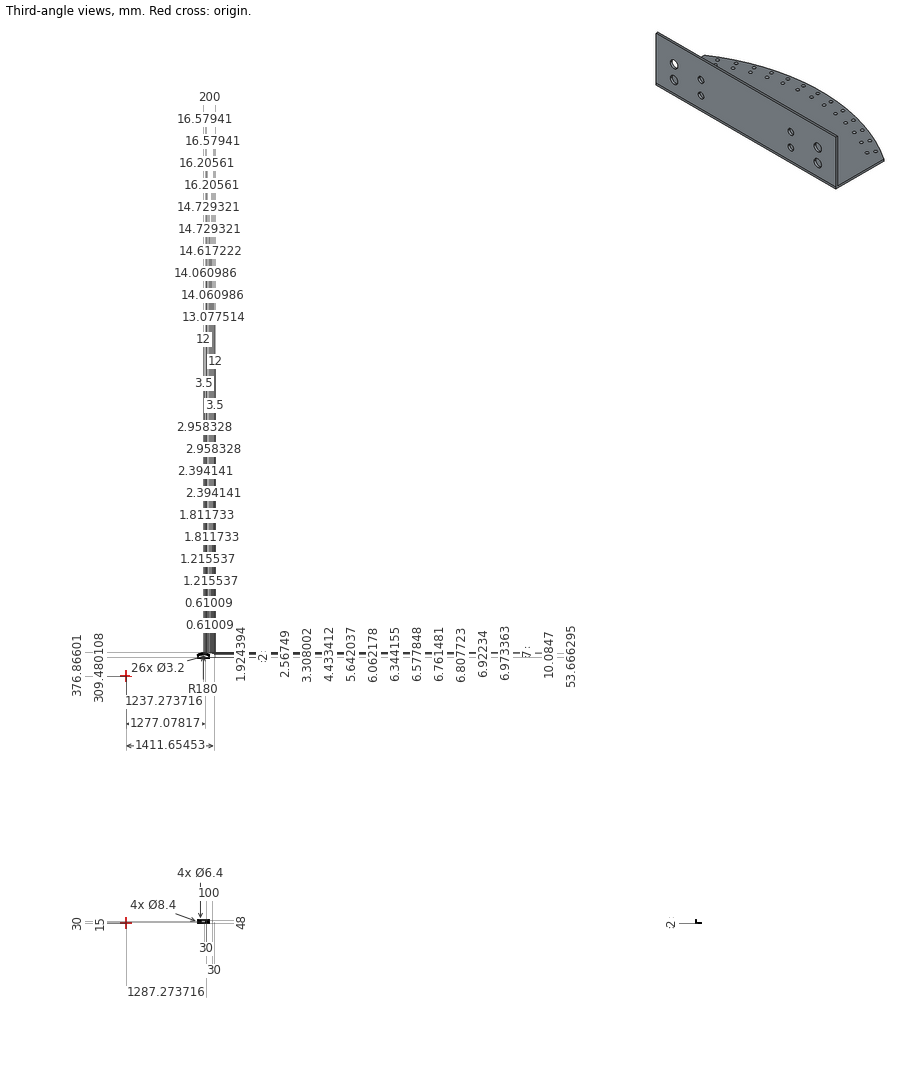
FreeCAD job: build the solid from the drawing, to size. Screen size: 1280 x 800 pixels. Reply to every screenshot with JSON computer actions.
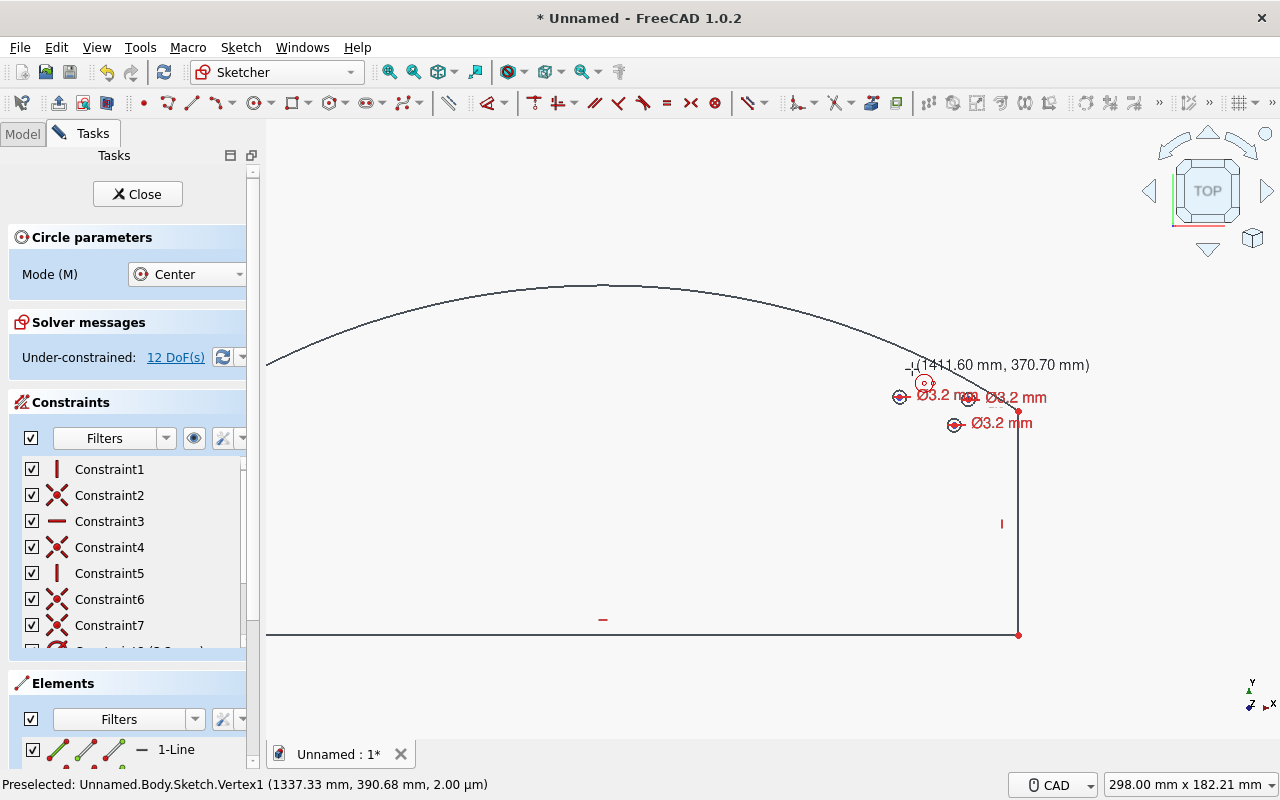
{"action": "left_click", "coordinate": [912, 369]}
{"action": "mouse_move", "coordinate": [907, 364]}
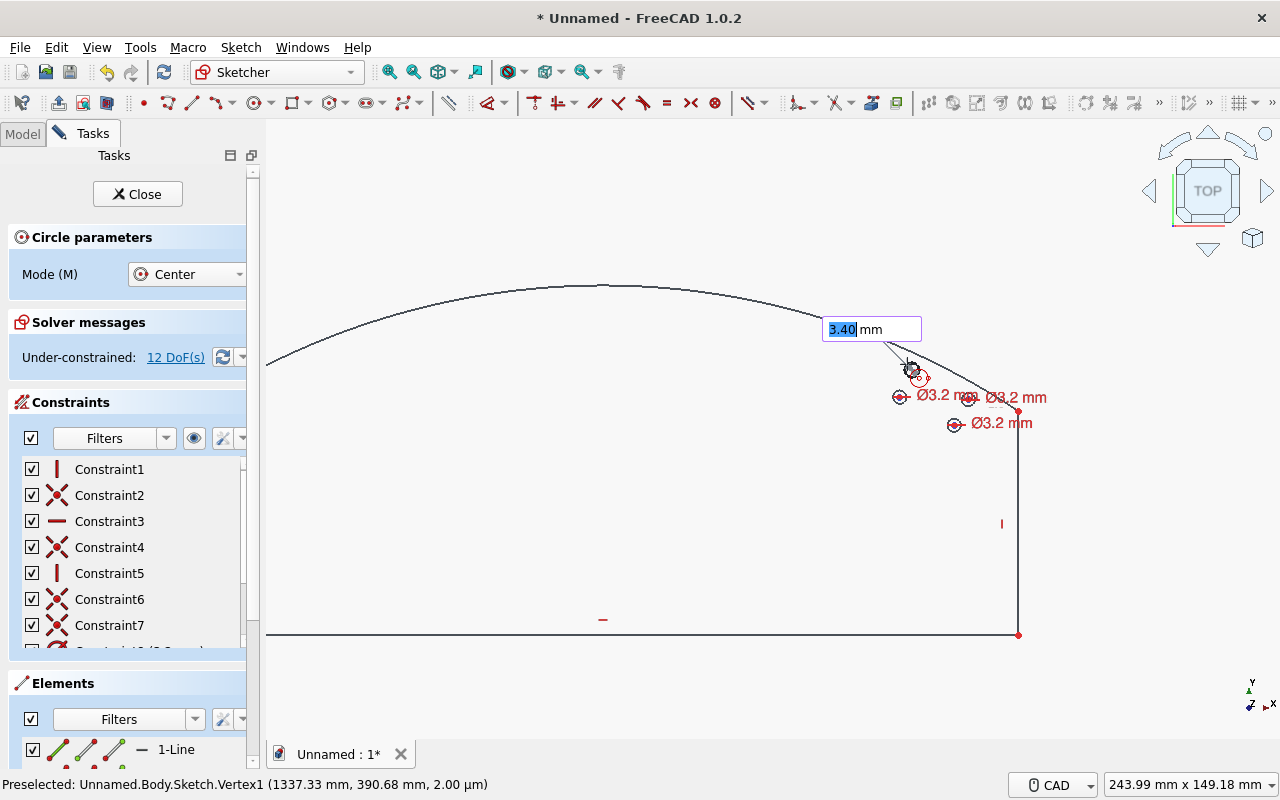
{"action": "type", "text": "3.2"}
{"action": "key", "text": "Return"}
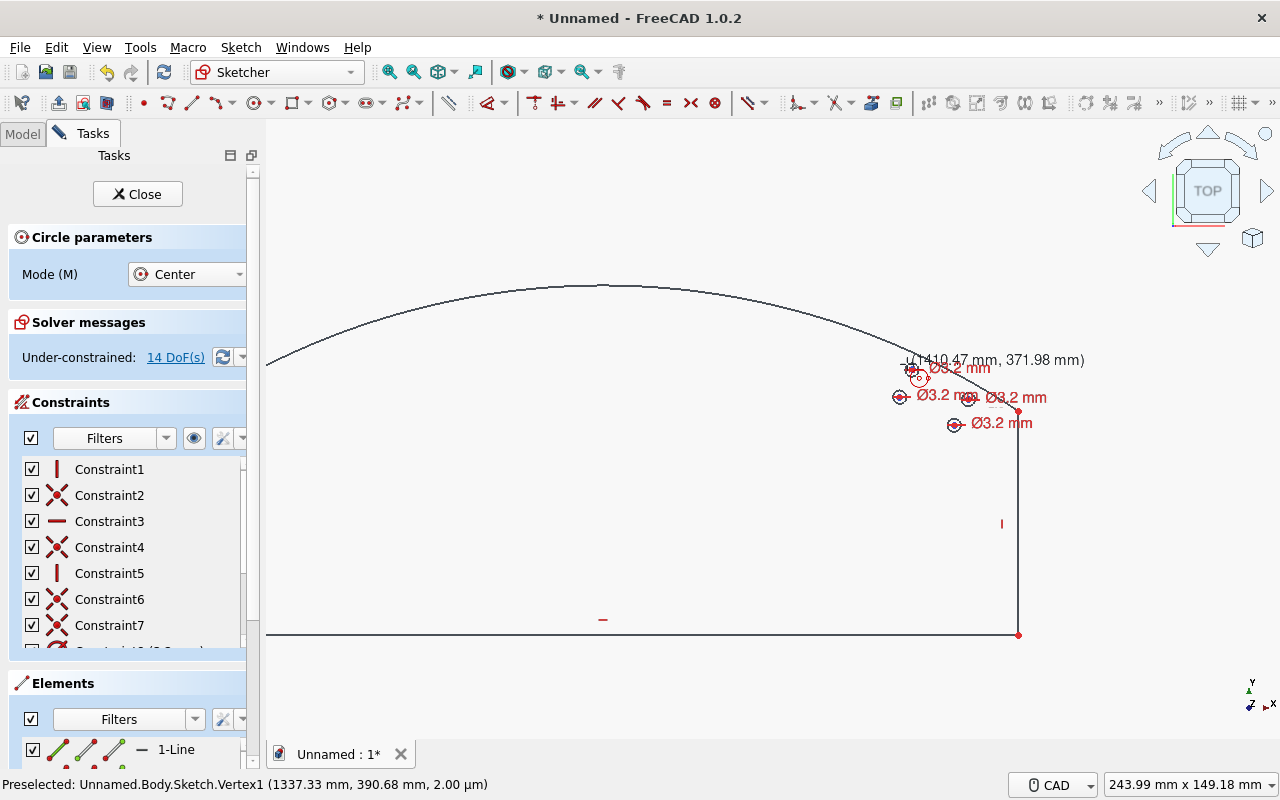
{"action": "scroll", "coordinate": [843, 372], "scroll_direction": "up", "scroll_amount": 7}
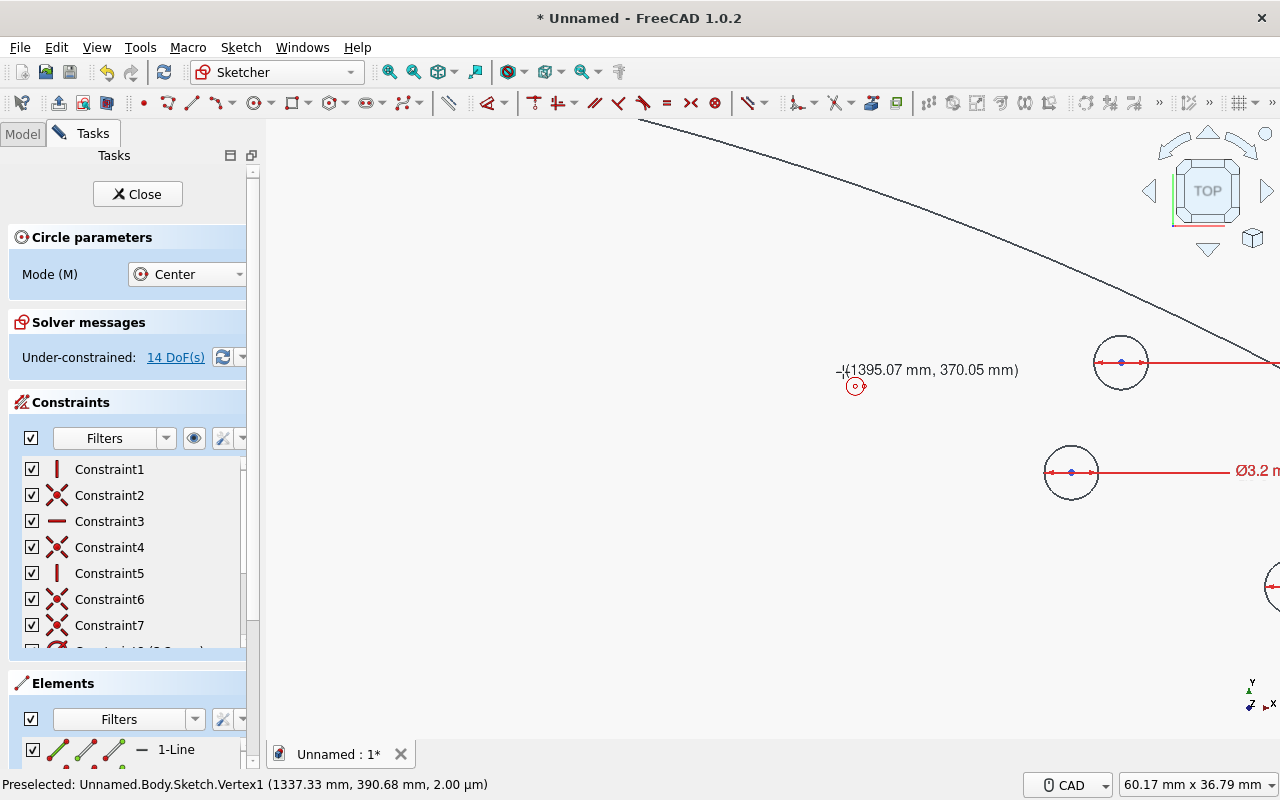
{"action": "scroll", "coordinate": [870, 371], "scroll_direction": "down", "scroll_amount": 9}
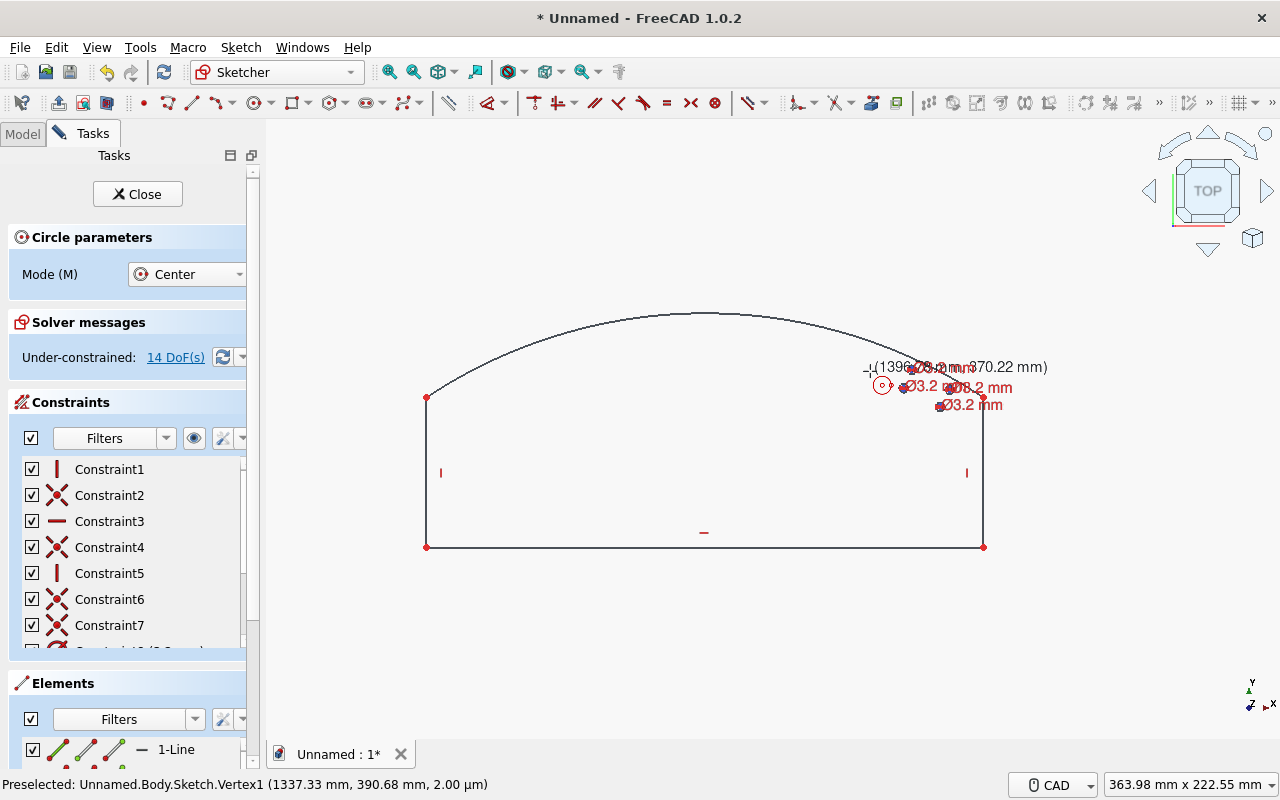
{"action": "left_click", "coordinate": [866, 371]}
{"action": "mouse_move", "coordinate": [869, 368]}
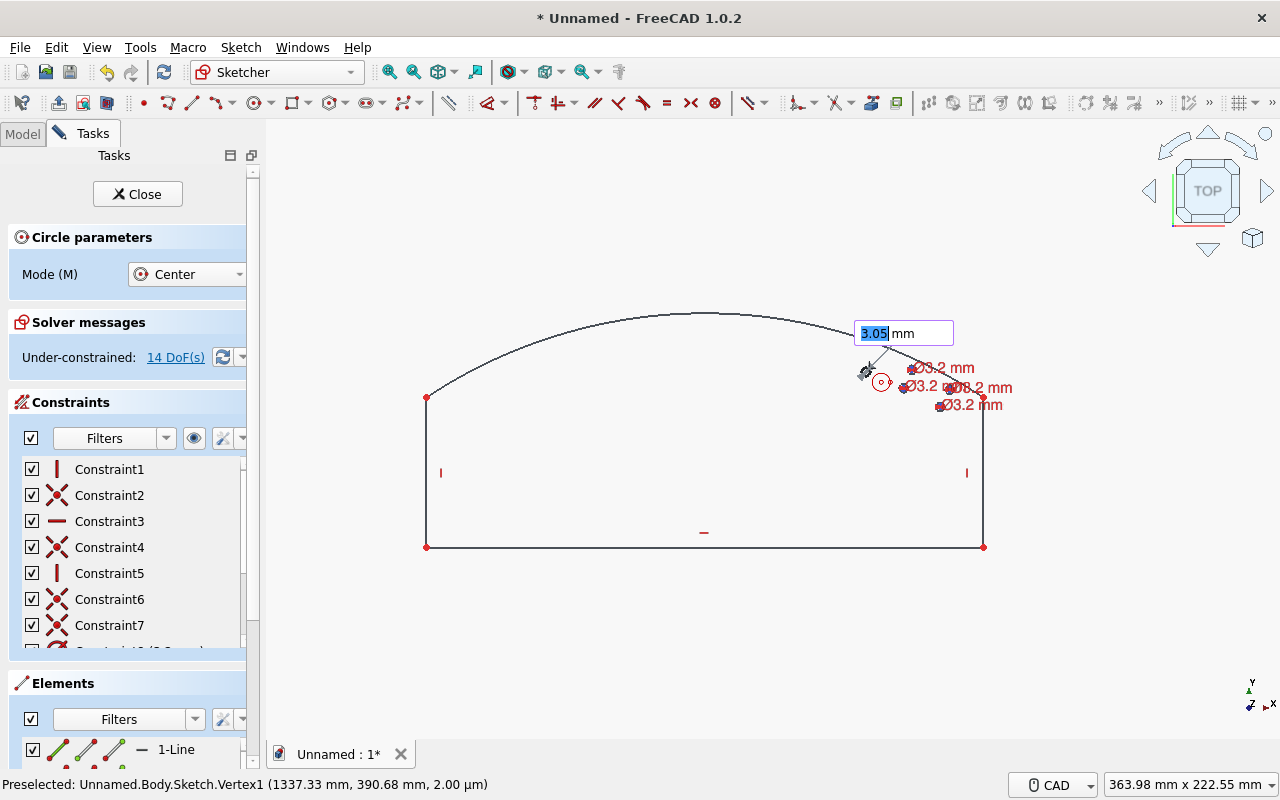
{"action": "type", "text": "3.2"}
{"action": "key", "text": "Return"}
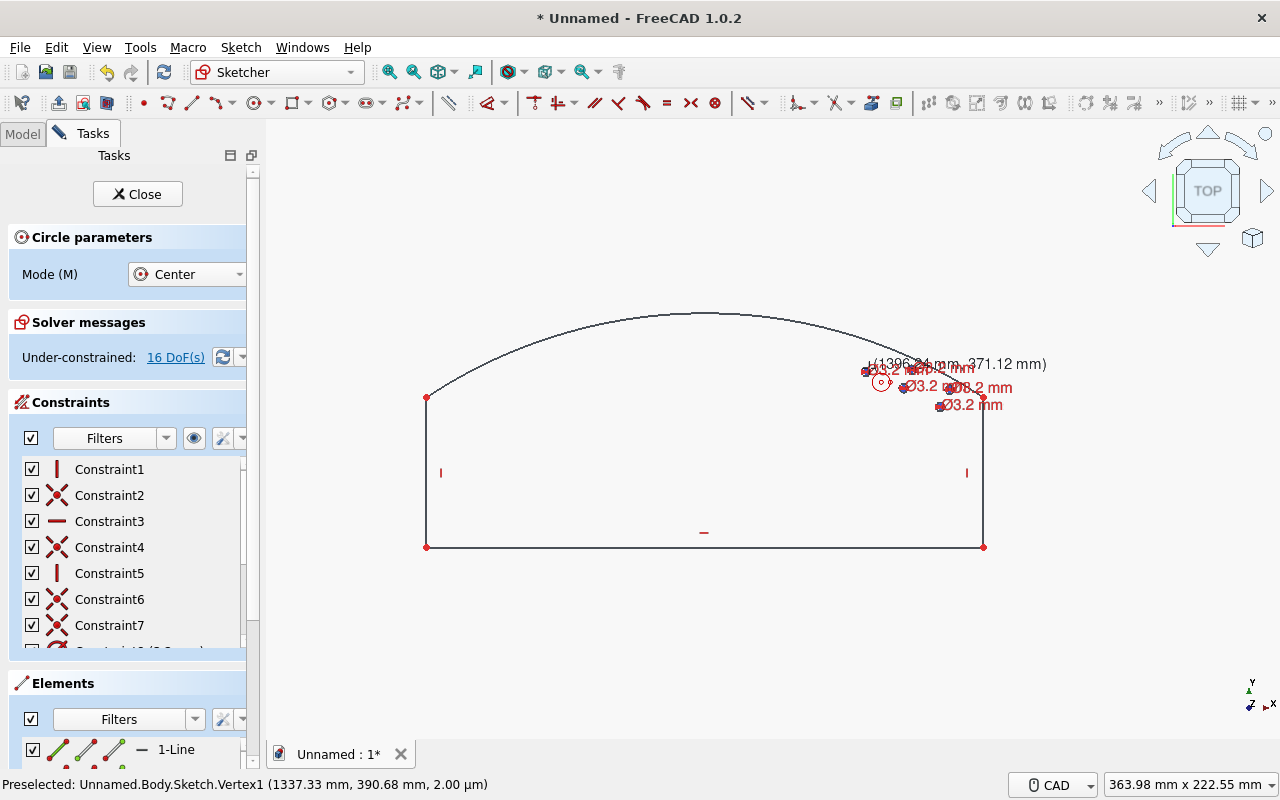
{"action": "scroll", "coordinate": [469, 406], "scroll_direction": "up", "scroll_amount": 9}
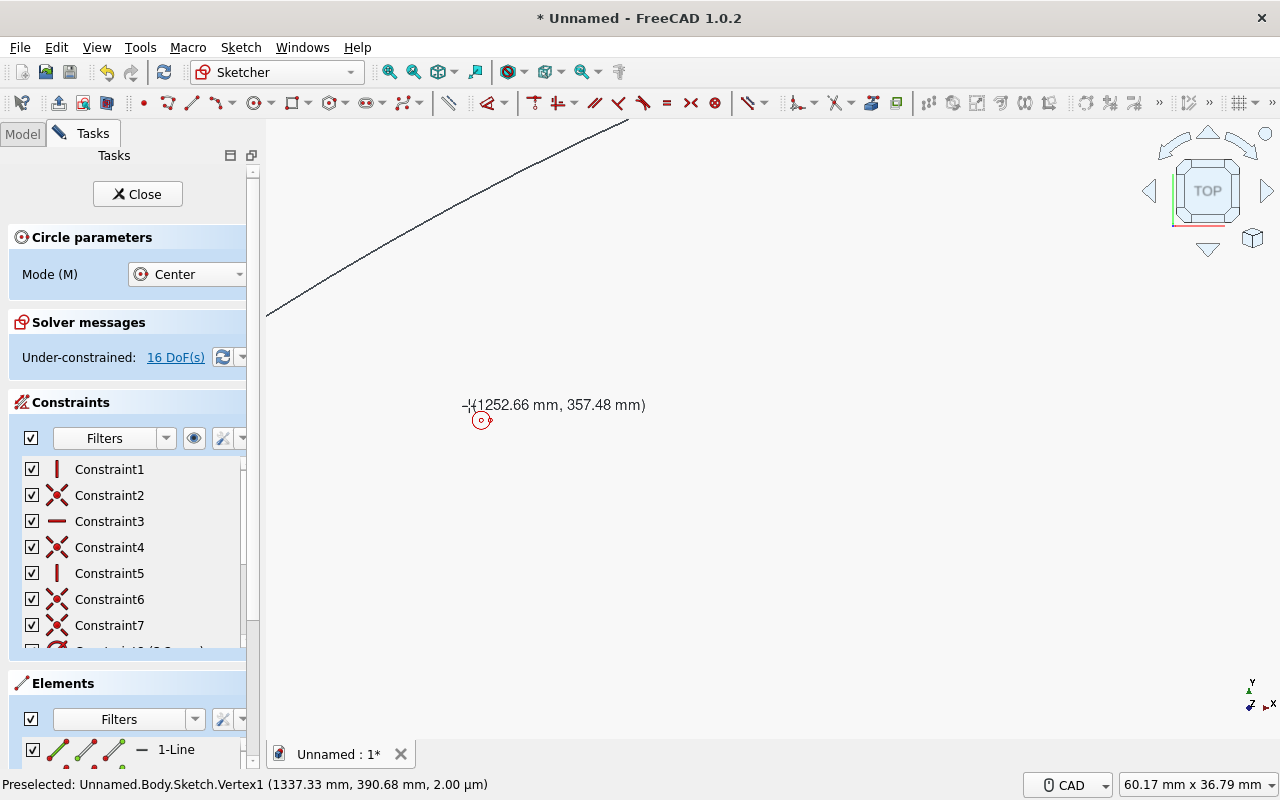
{"action": "scroll", "coordinate": [469, 406], "scroll_direction": "down", "scroll_amount": 9}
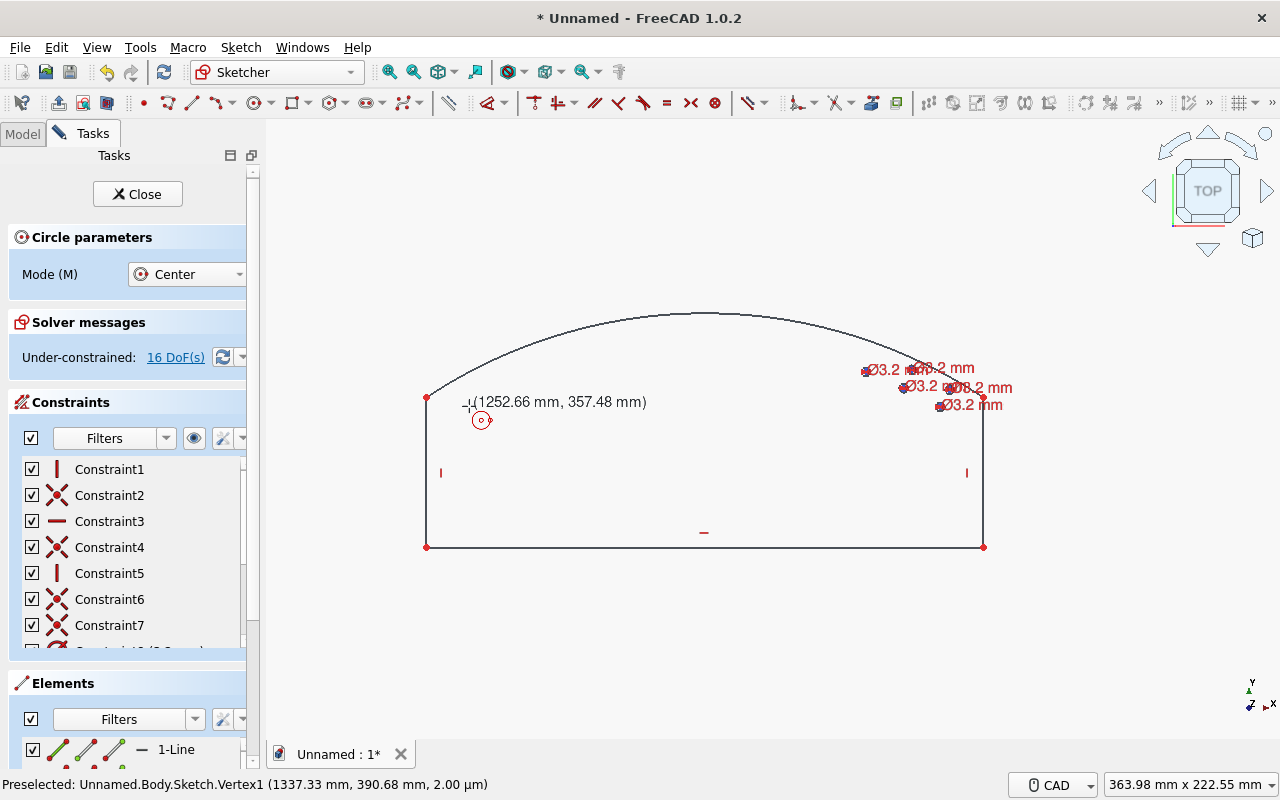
{"action": "left_click", "coordinate": [469, 406]}
{"action": "mouse_move", "coordinate": [472, 403]}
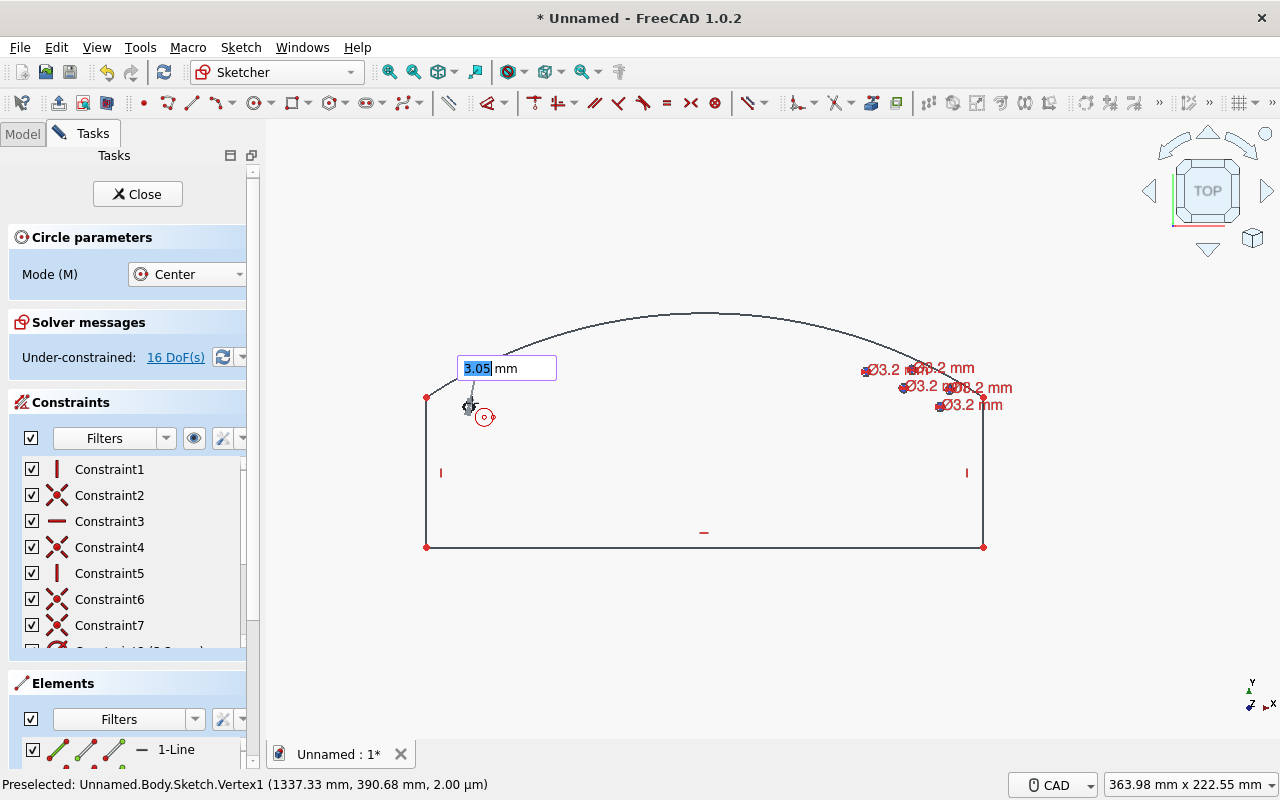
{"action": "type", "text": "3.2"}
{"action": "key", "text": "Return"}